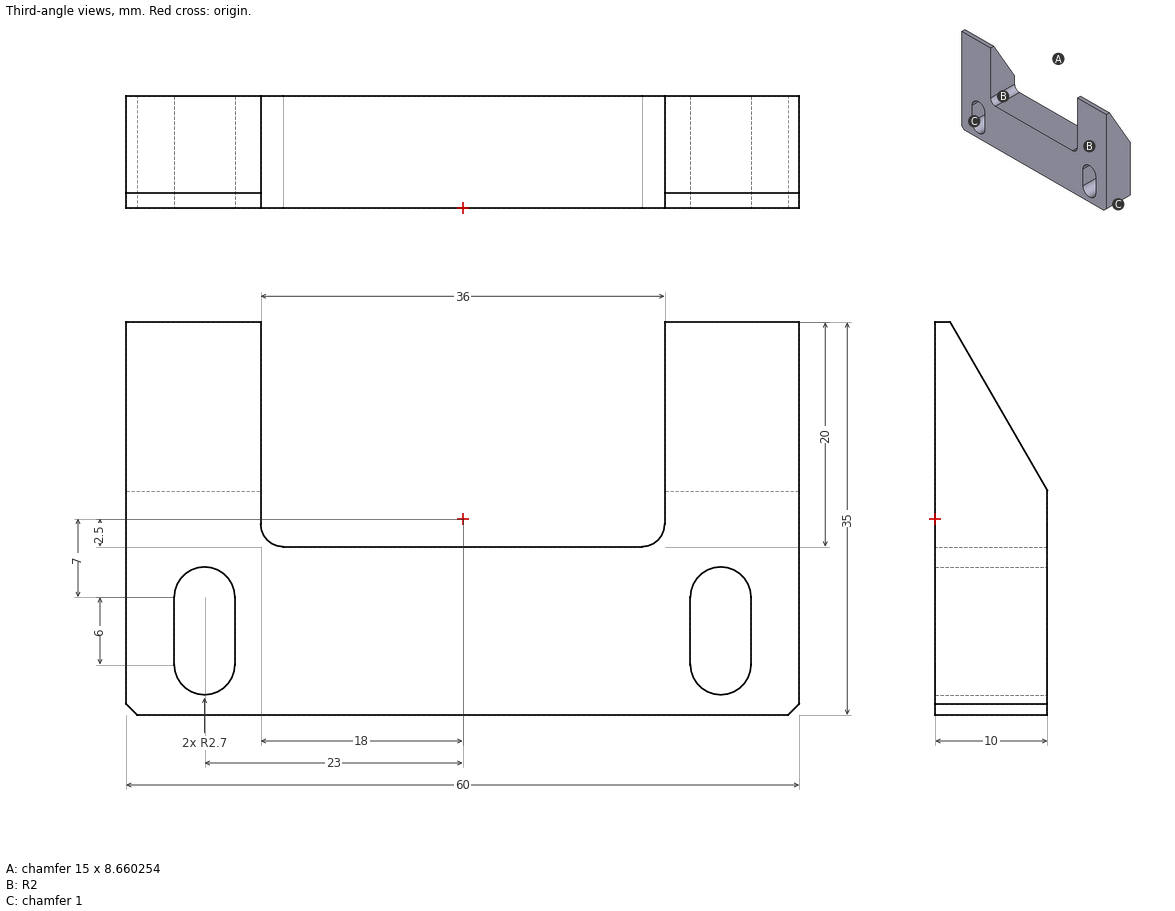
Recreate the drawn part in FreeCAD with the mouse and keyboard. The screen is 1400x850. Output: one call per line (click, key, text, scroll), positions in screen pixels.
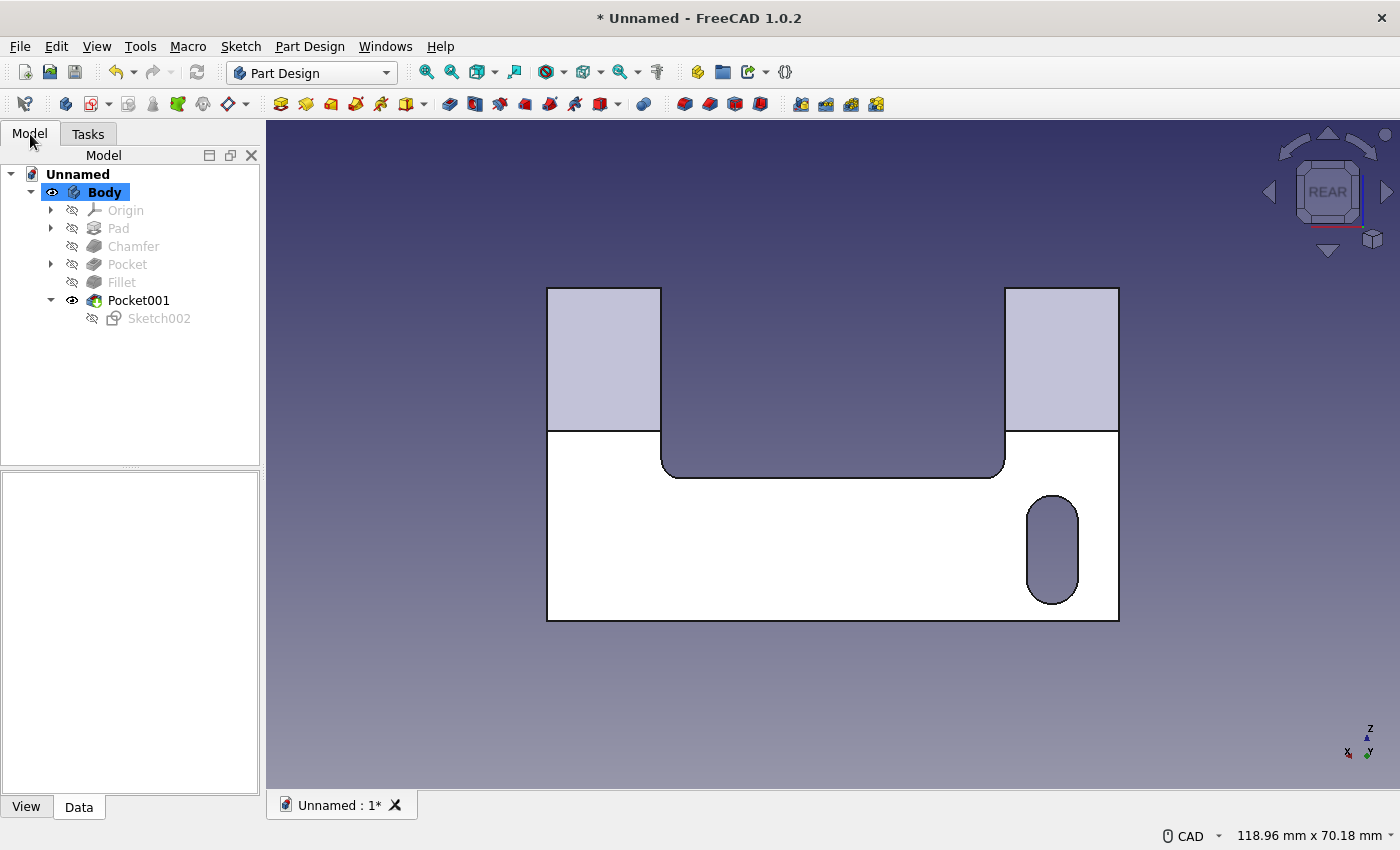
click(117, 300)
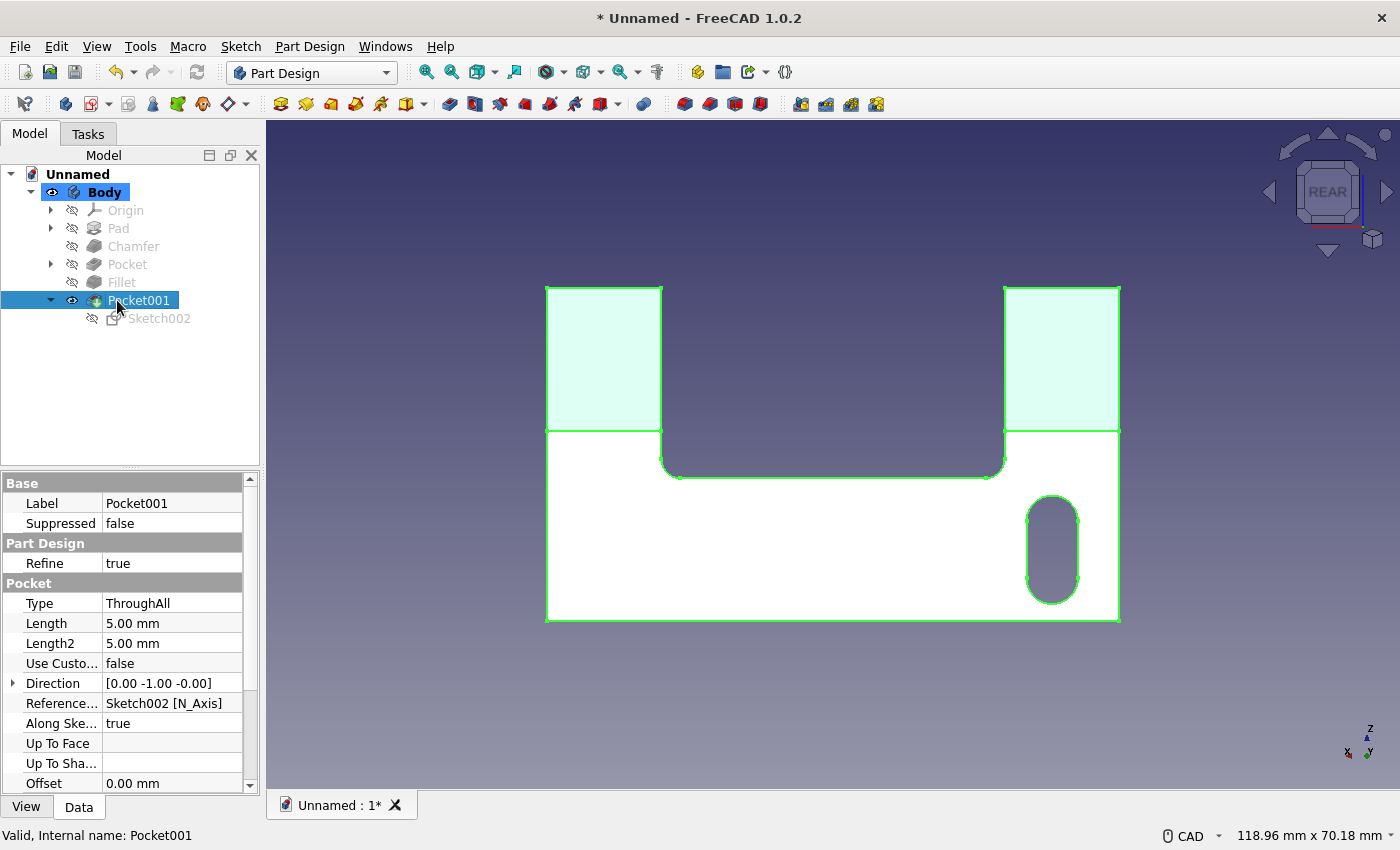
click(801, 104)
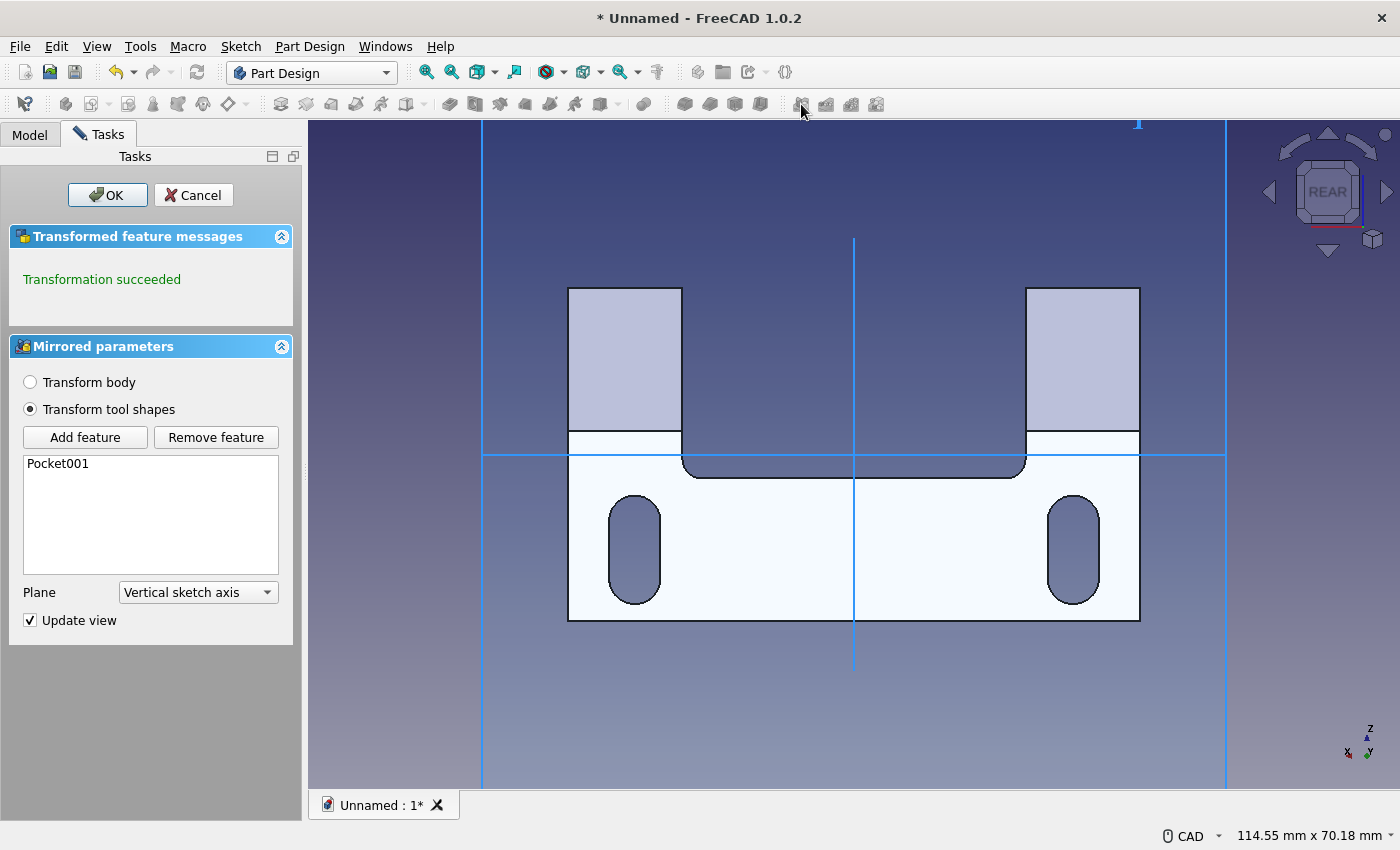
click(199, 592)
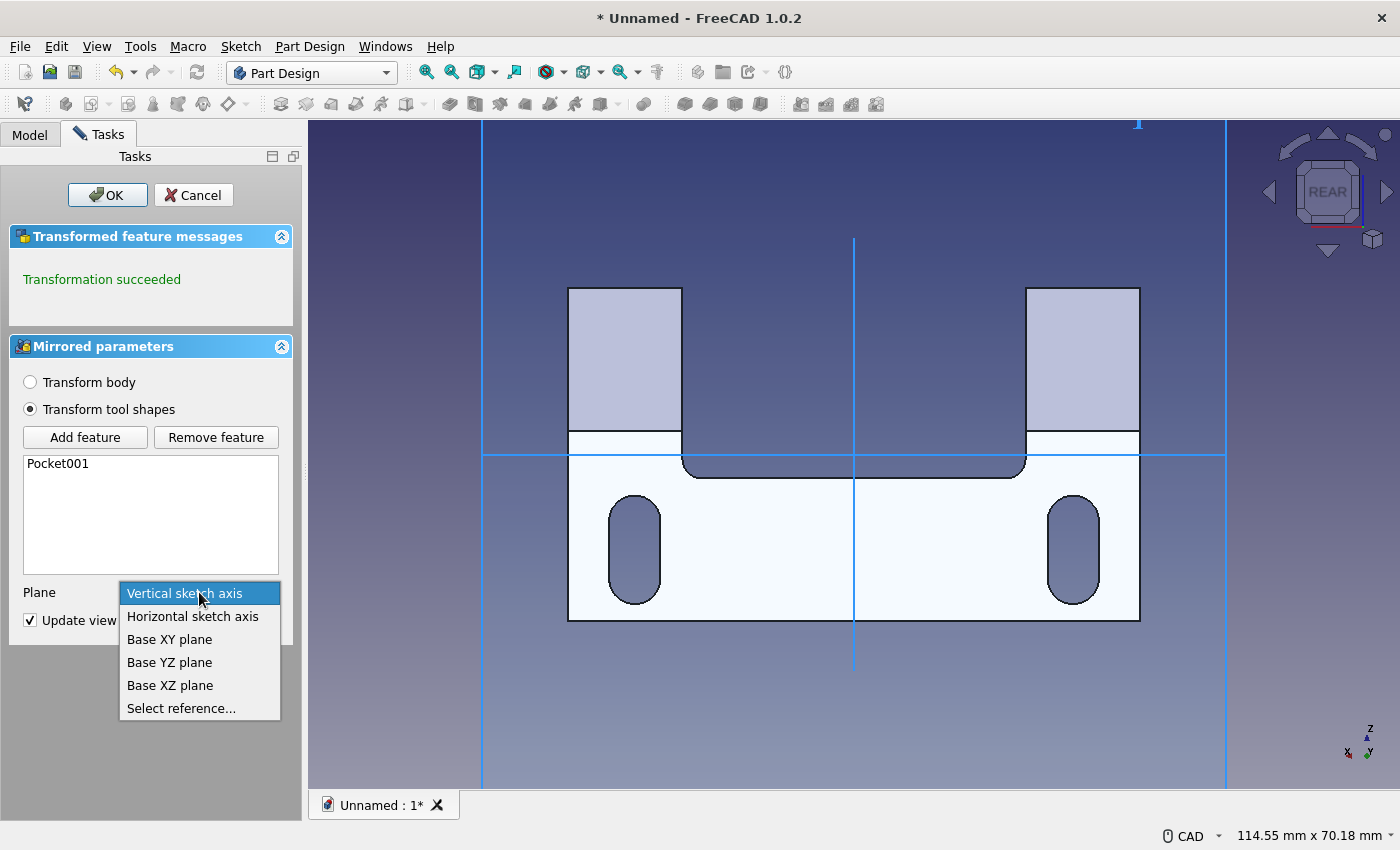
click(198, 662)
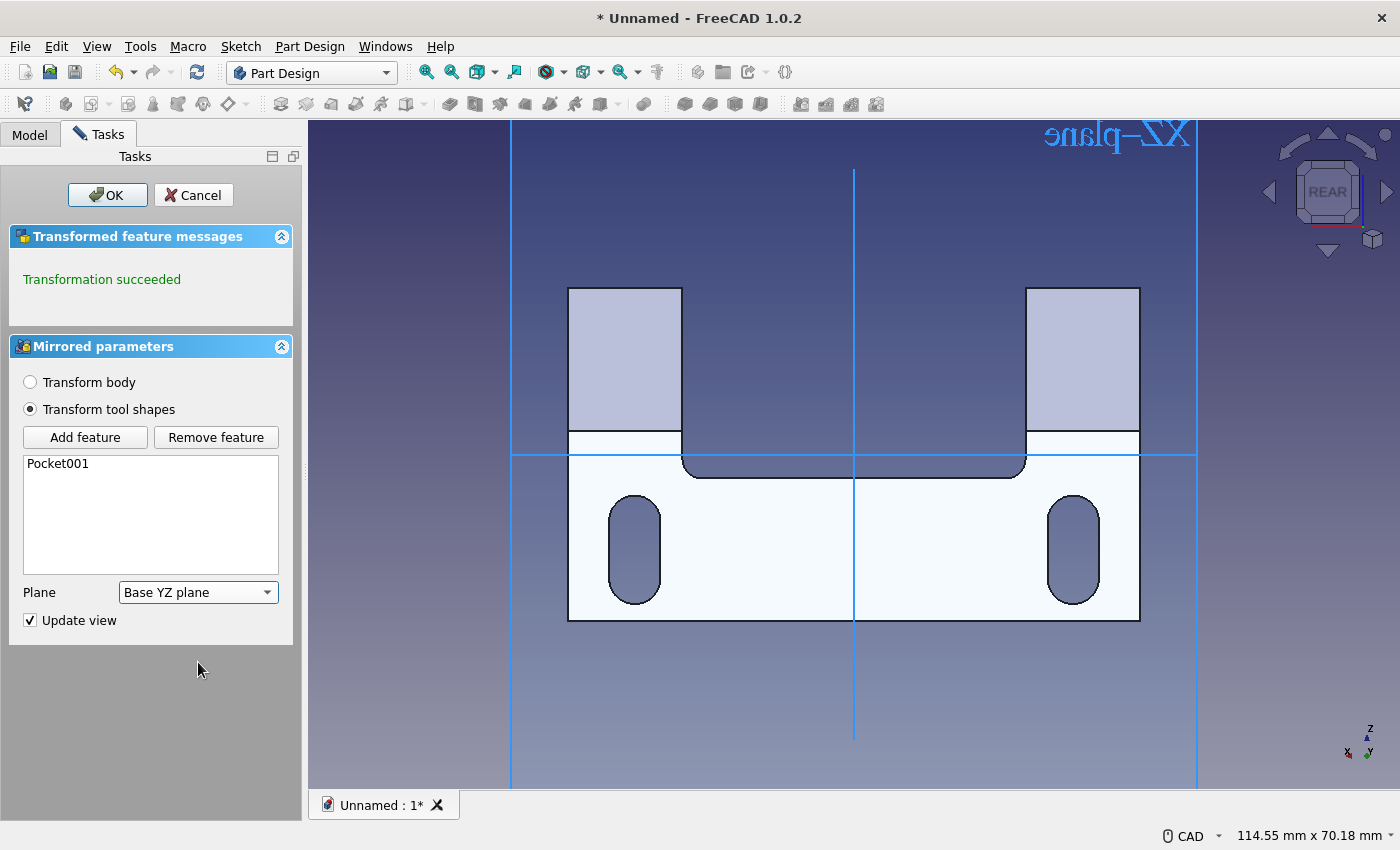
click(108, 195)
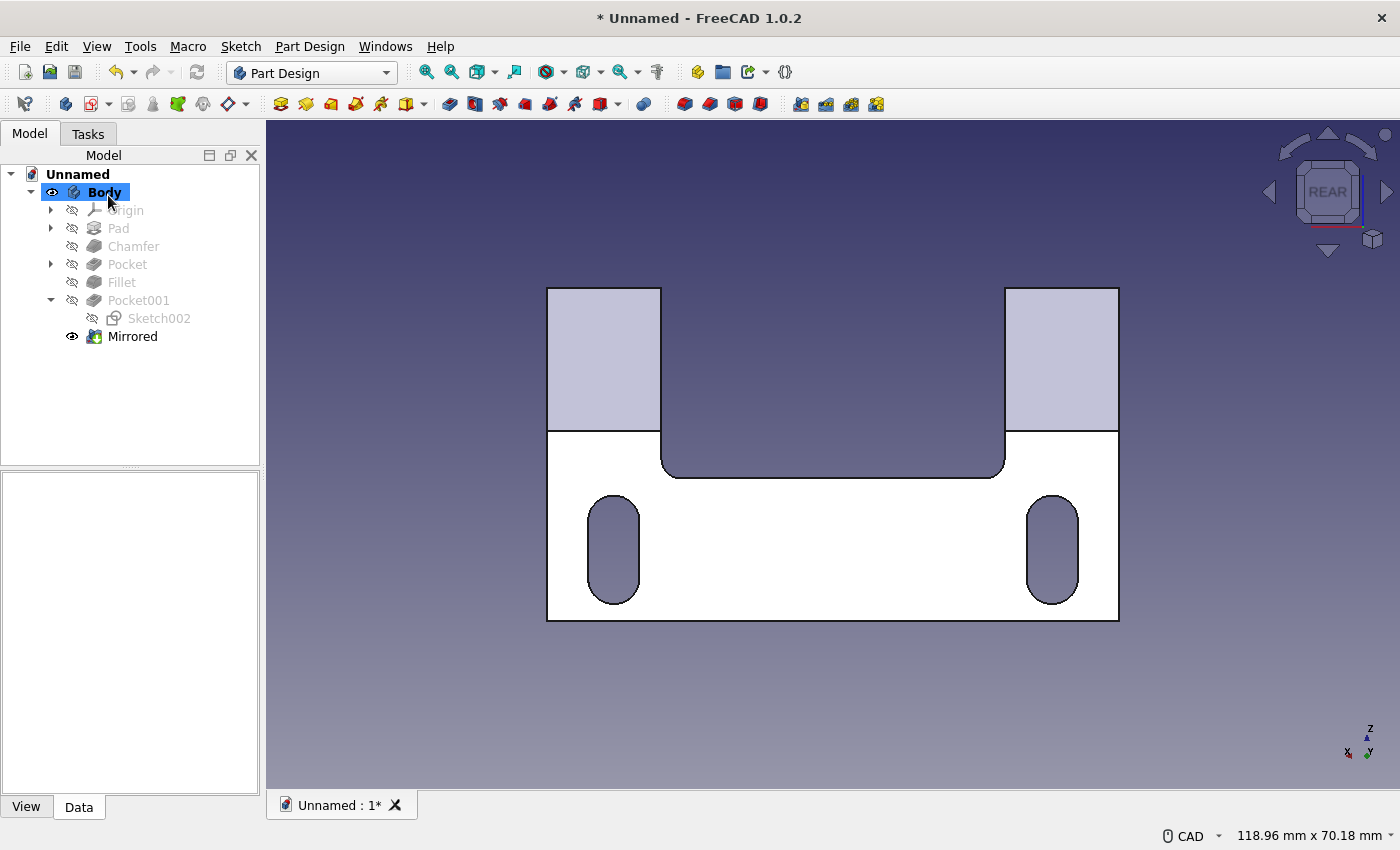
key(0)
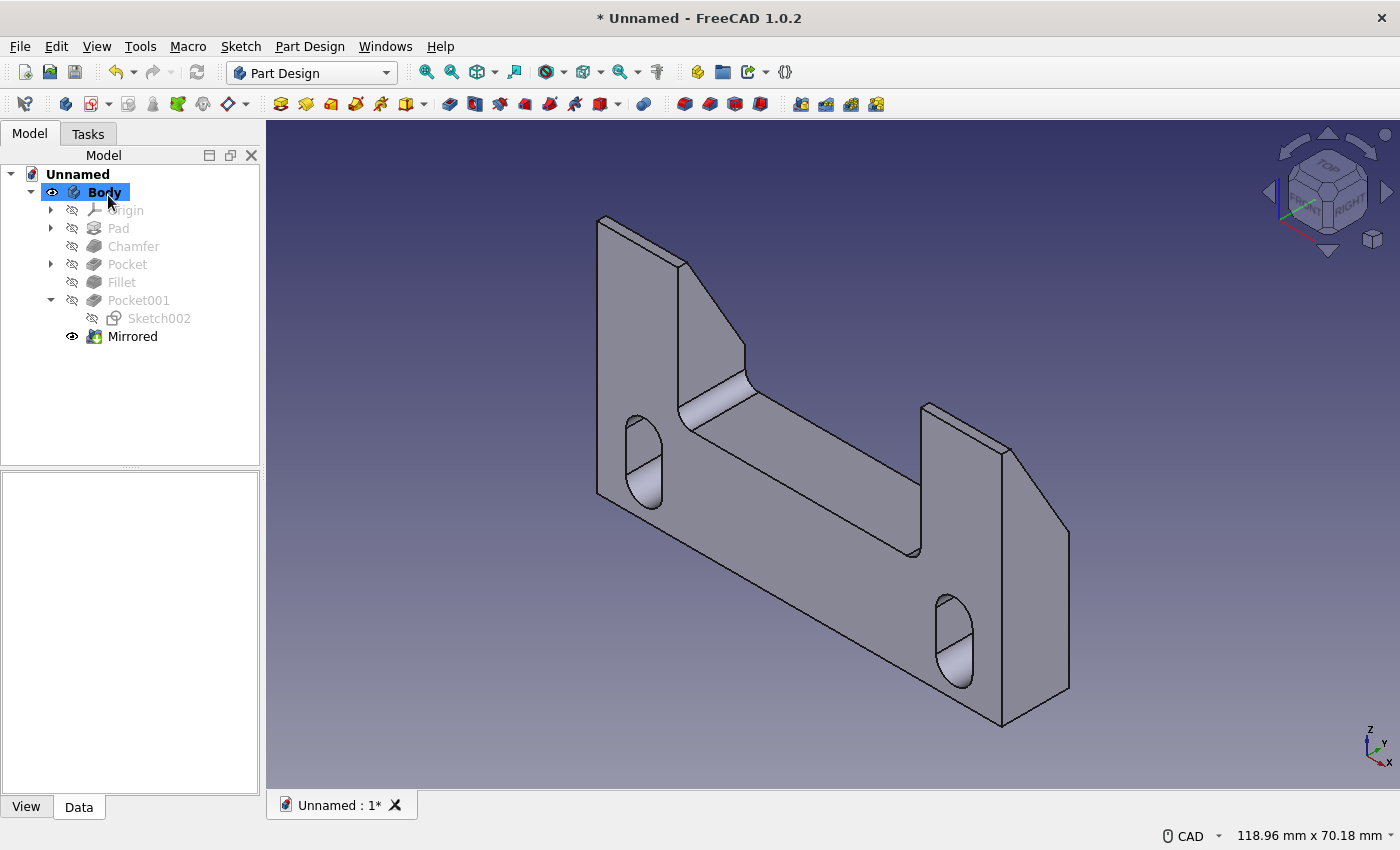
key(2)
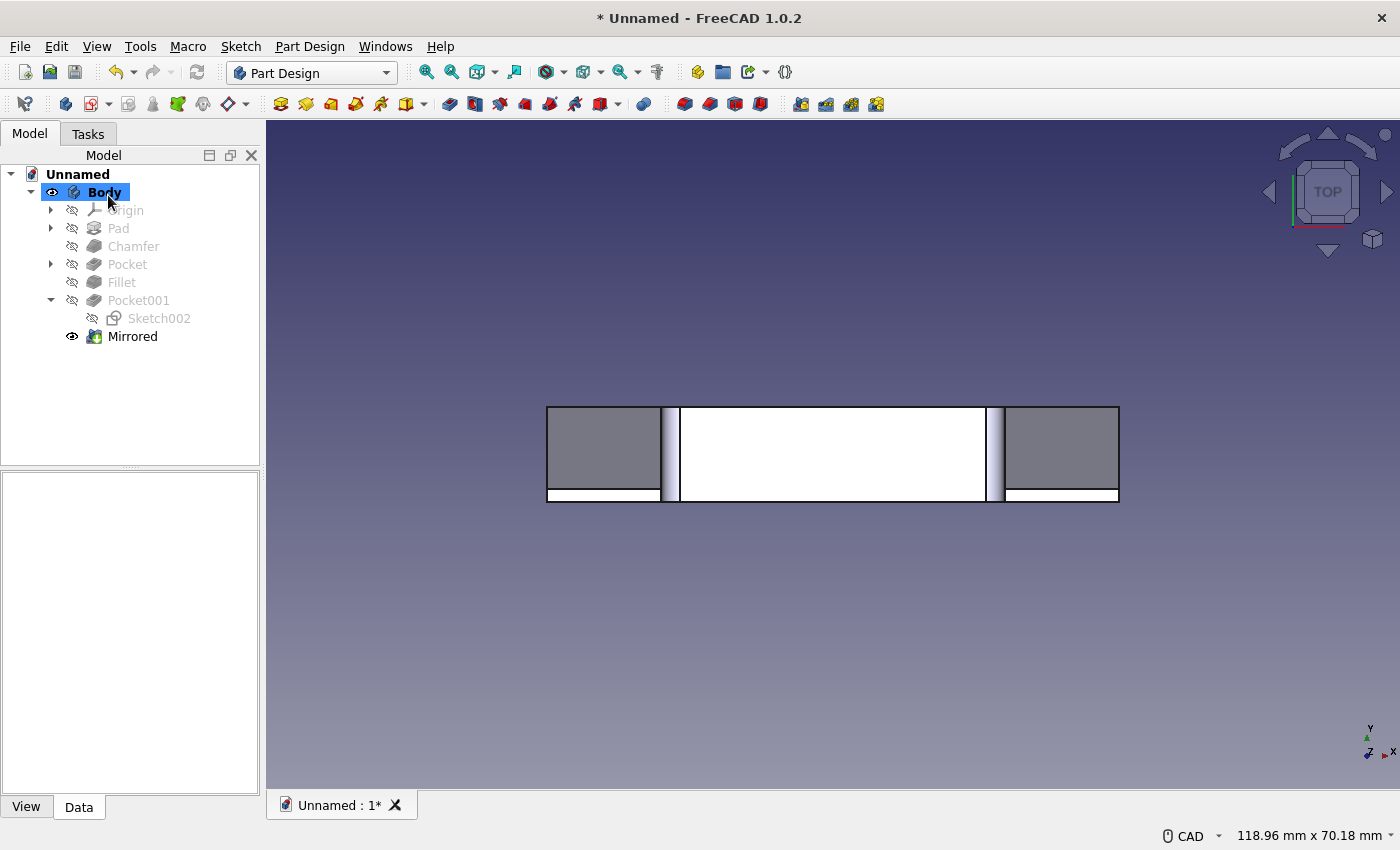
key(1)